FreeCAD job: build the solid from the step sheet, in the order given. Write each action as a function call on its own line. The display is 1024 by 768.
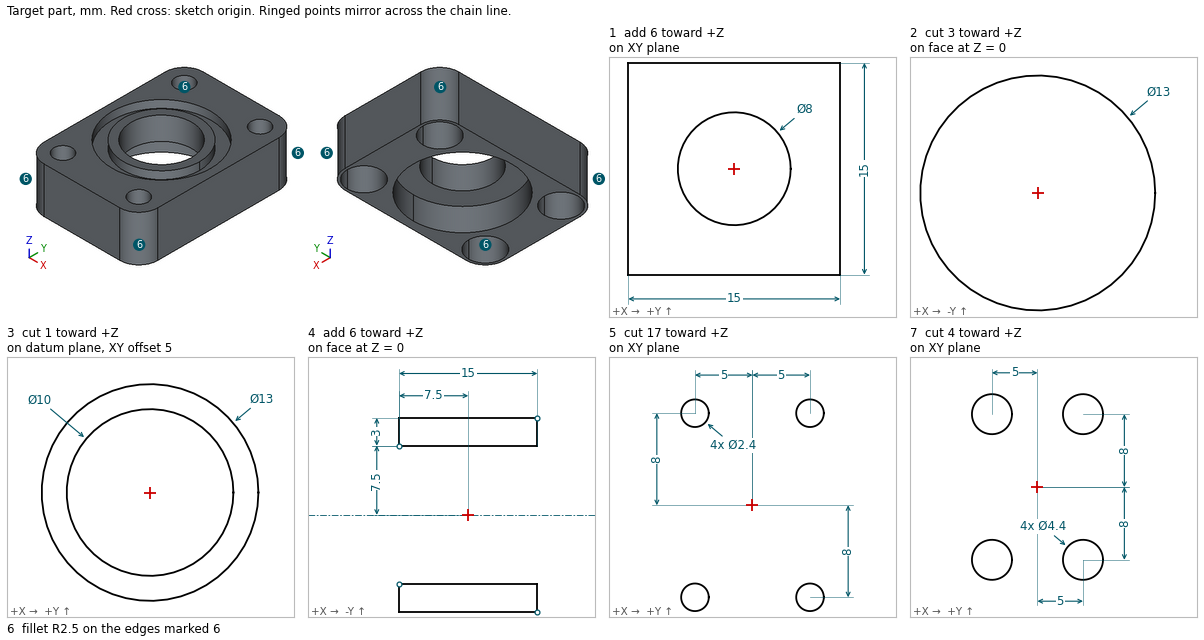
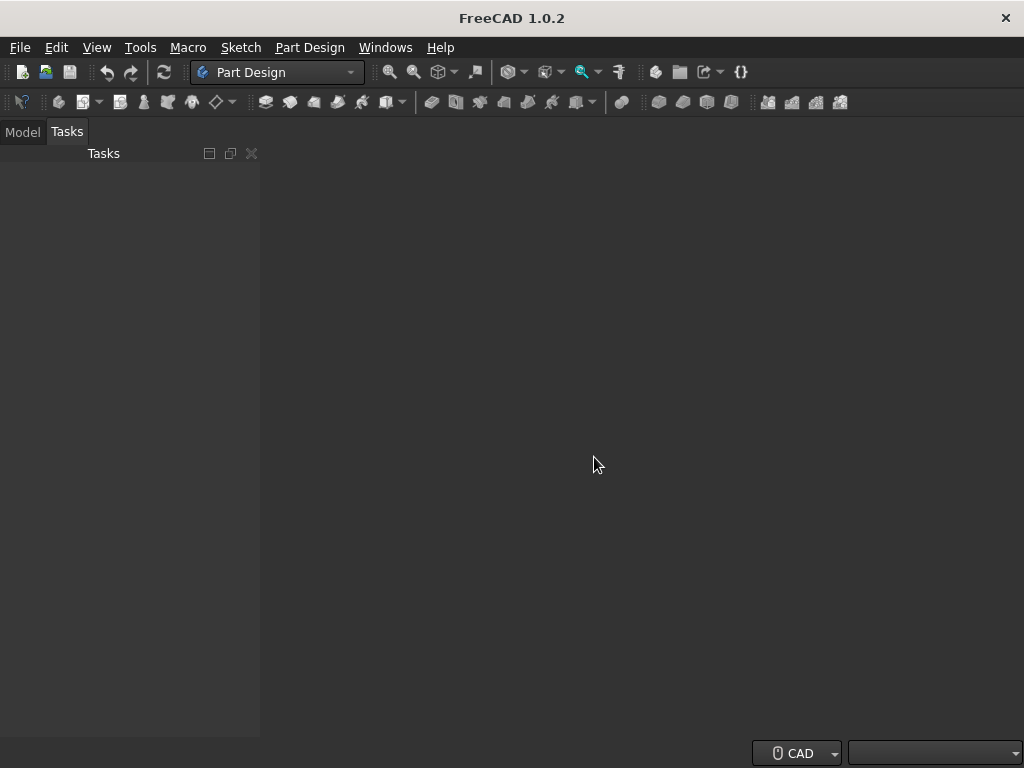
click(22, 72)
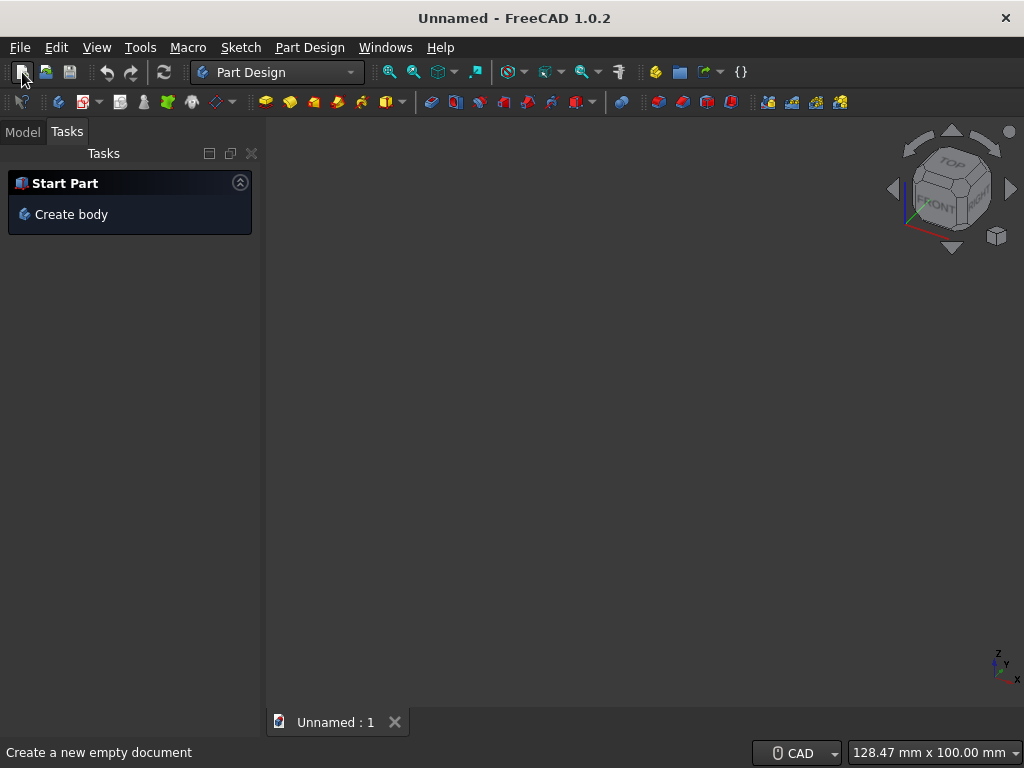
click(84, 102)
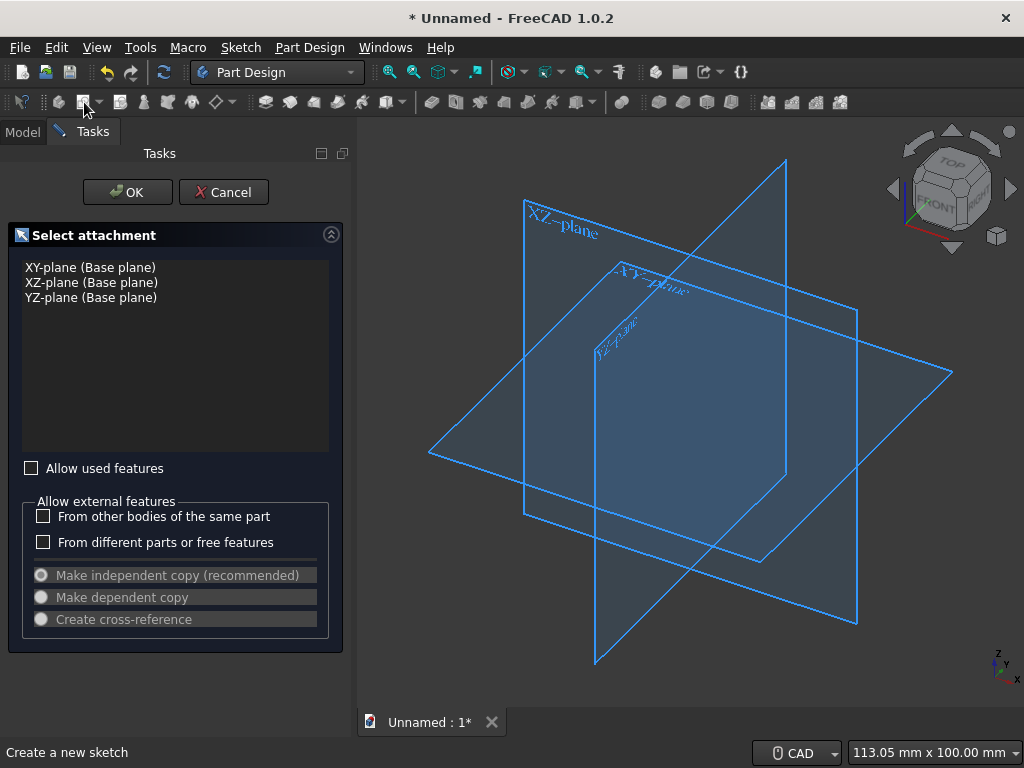
click(82, 268)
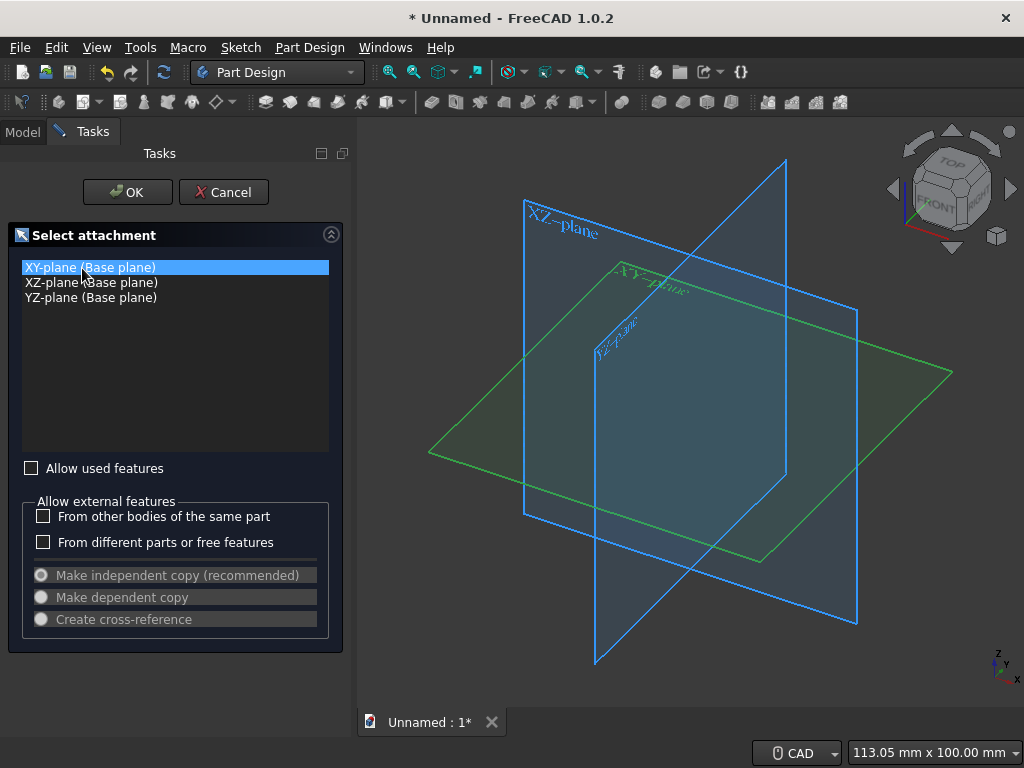
click(128, 192)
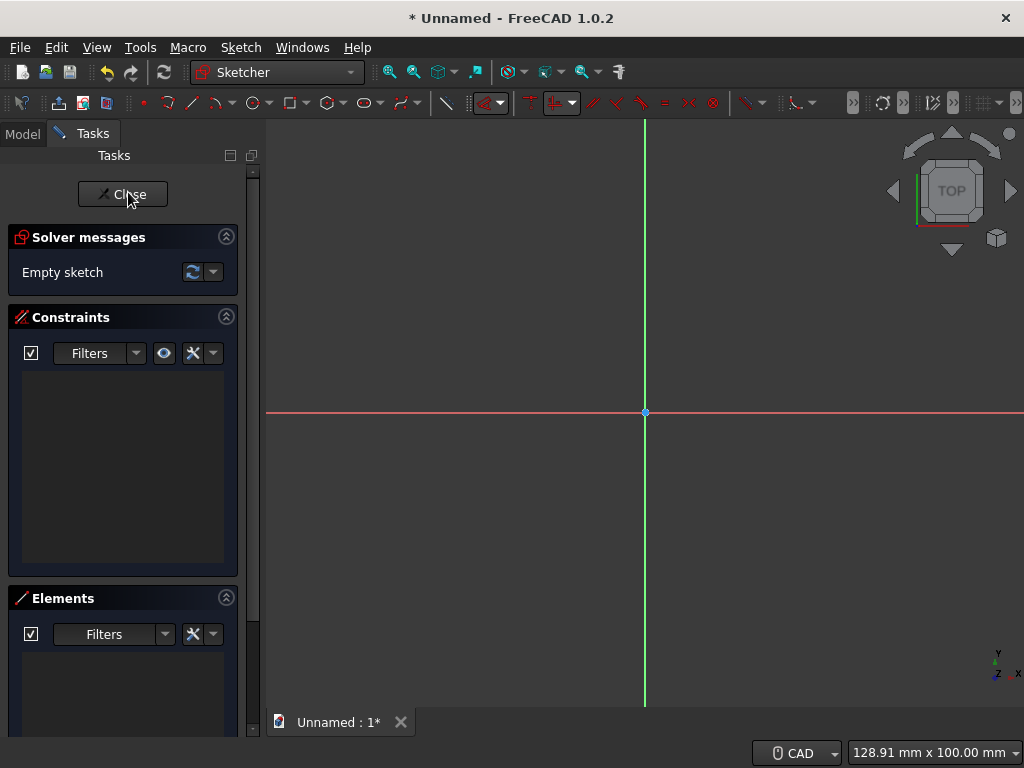
scroll(667, 413, up, 7)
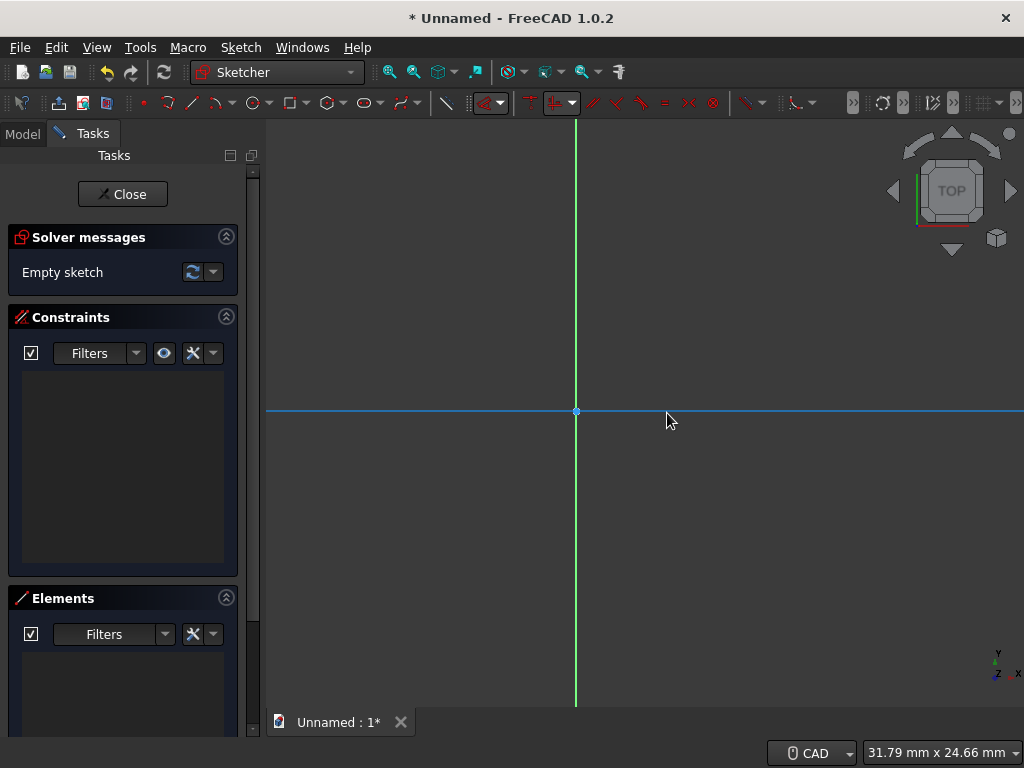
key(g)
key(v)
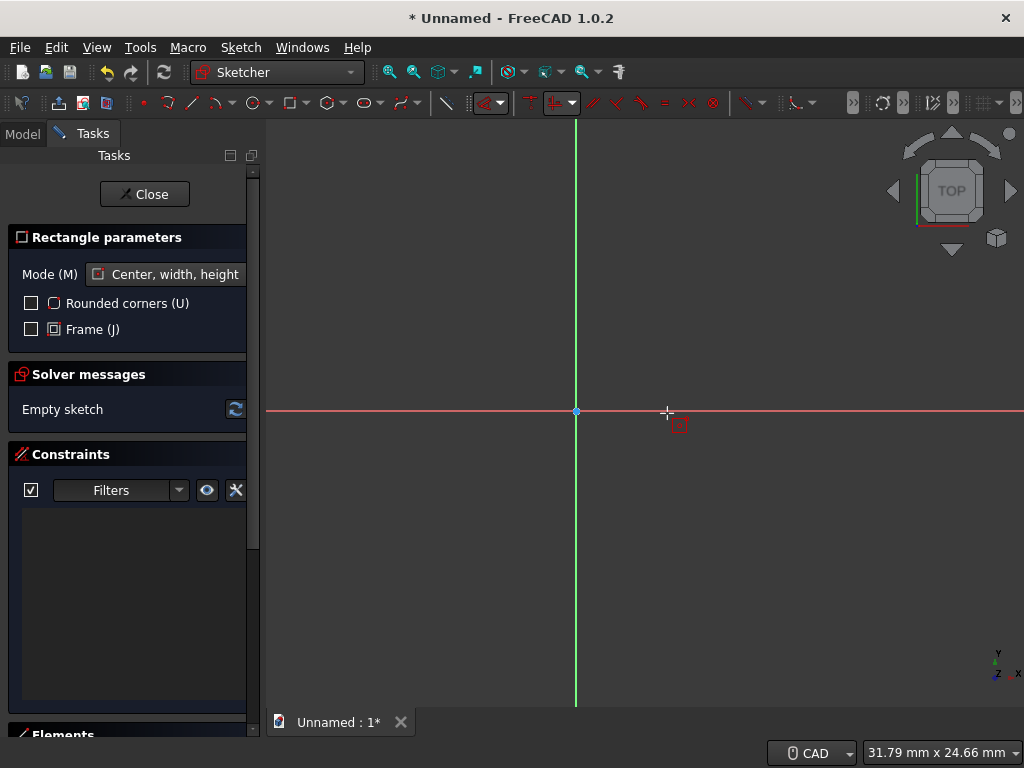
click(576, 411)
click(755, 233)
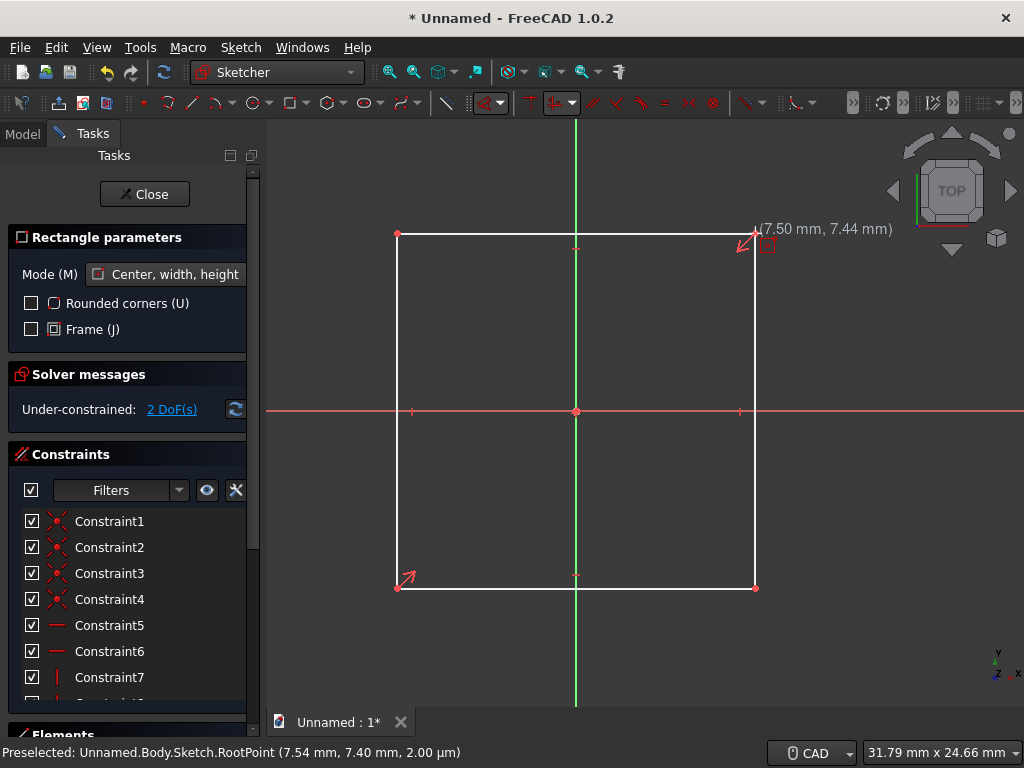
key(g)
key(c)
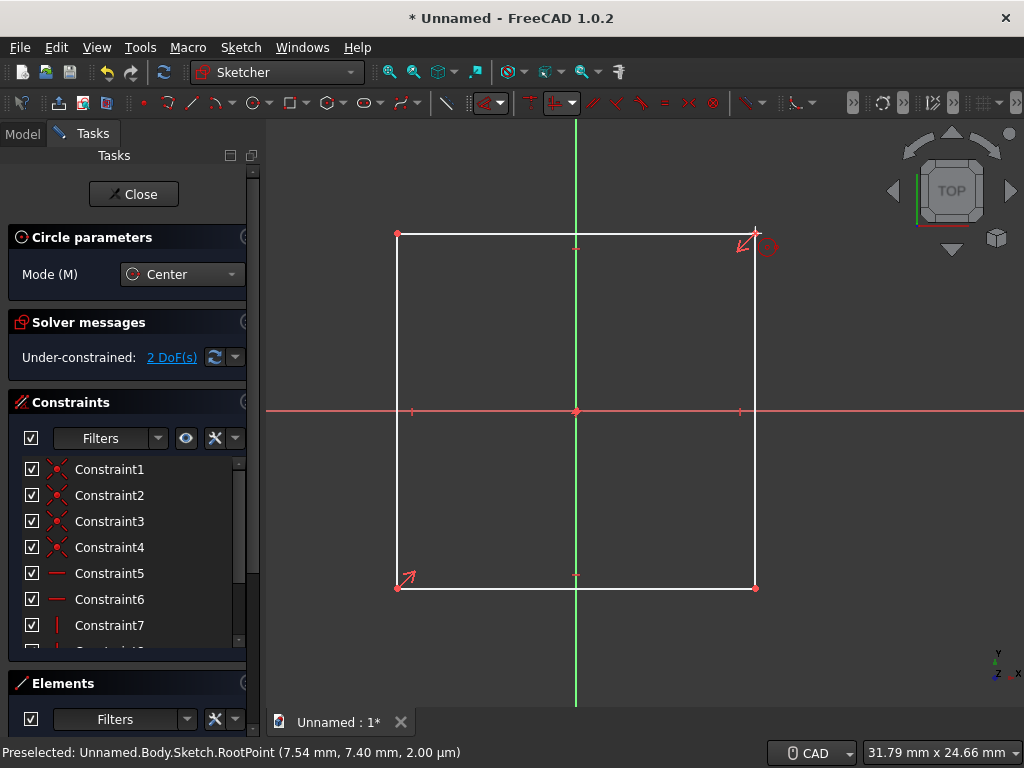
click(576, 411)
click(644, 344)
key(Escape)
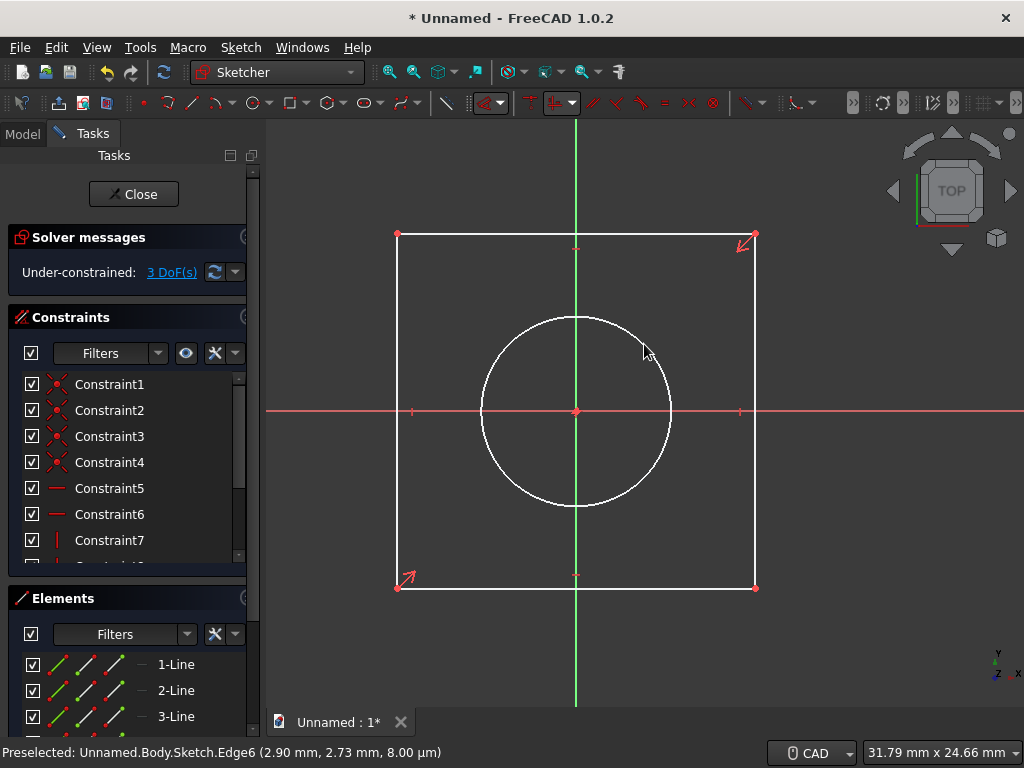
key(d)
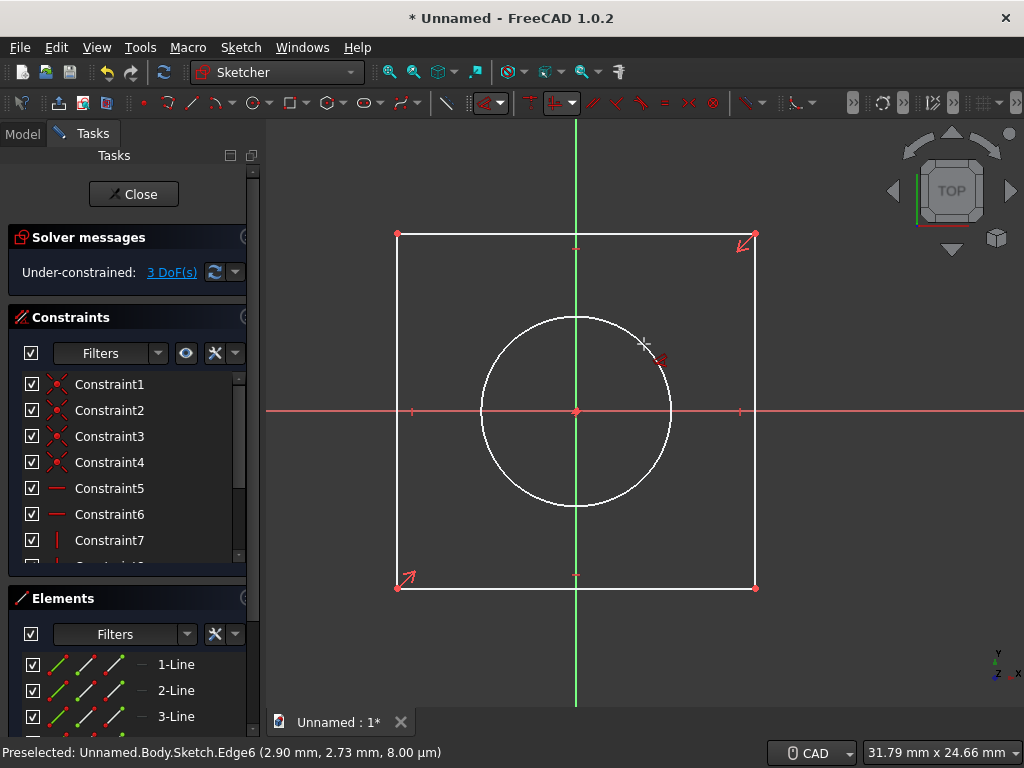
click(643, 344)
click(666, 321)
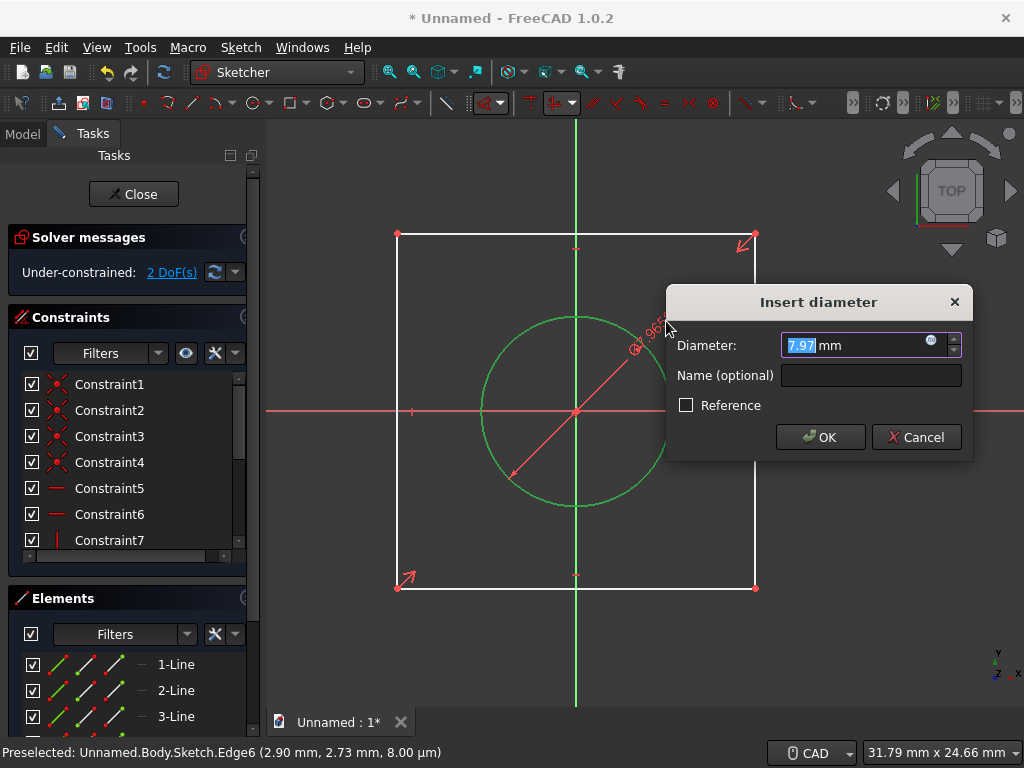
text(8)
key(Return)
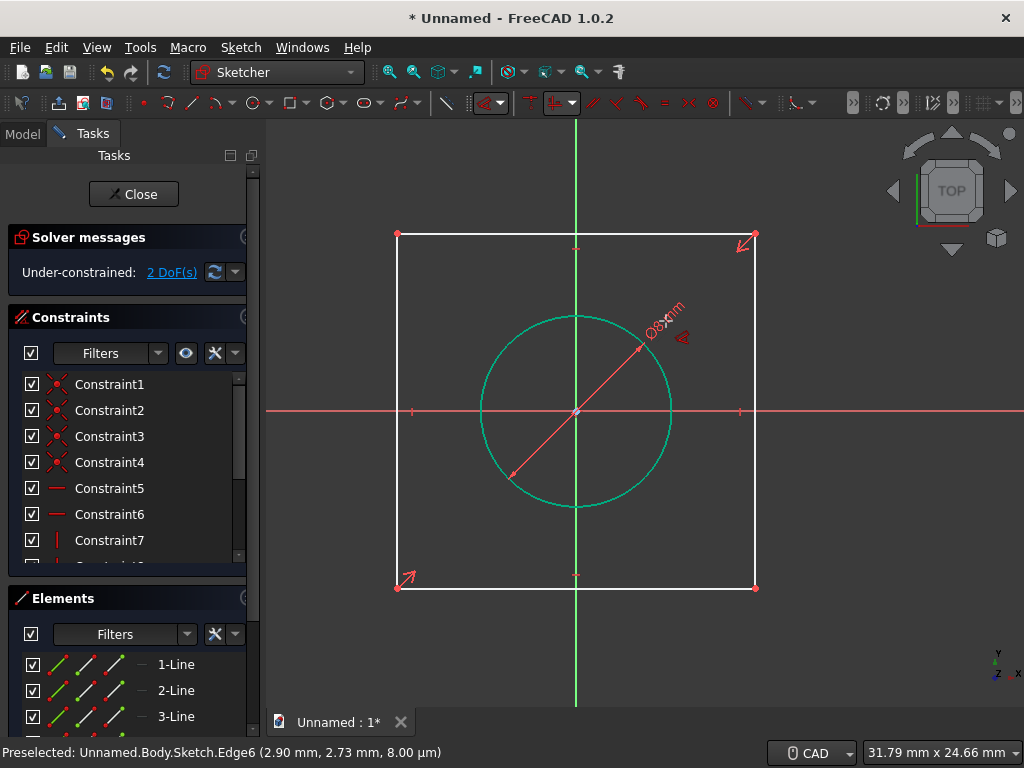
click(505, 589)
click(494, 623)